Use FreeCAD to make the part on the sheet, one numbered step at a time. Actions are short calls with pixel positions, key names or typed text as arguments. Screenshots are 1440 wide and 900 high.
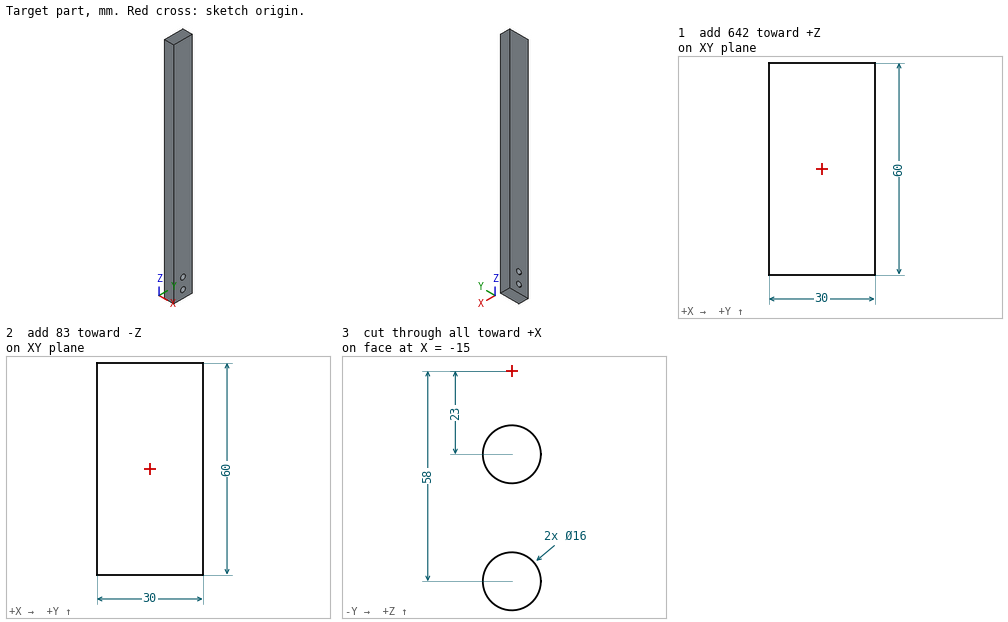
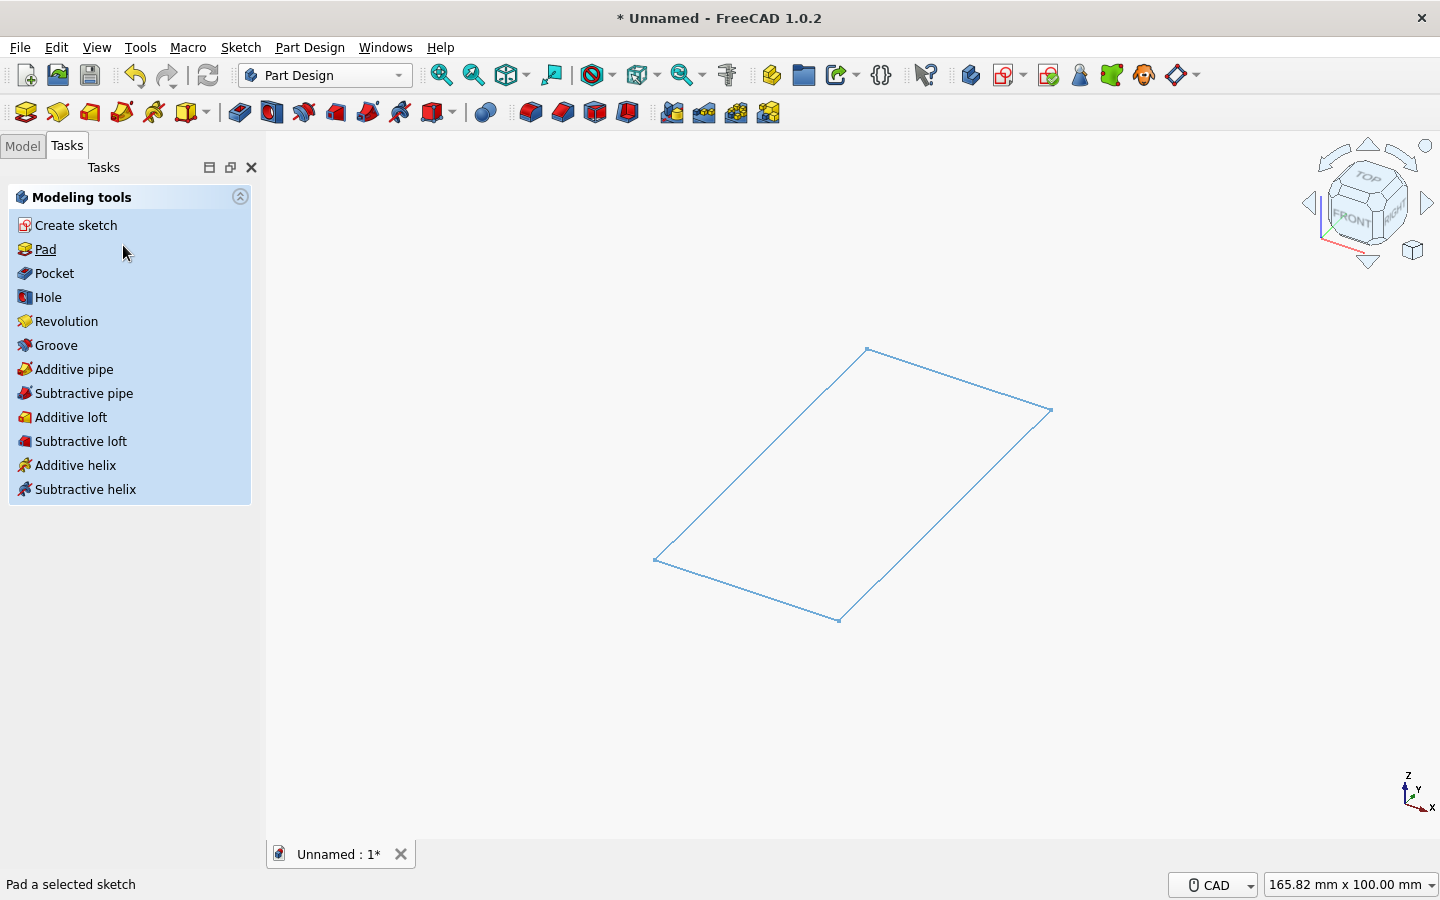
click(26, 112)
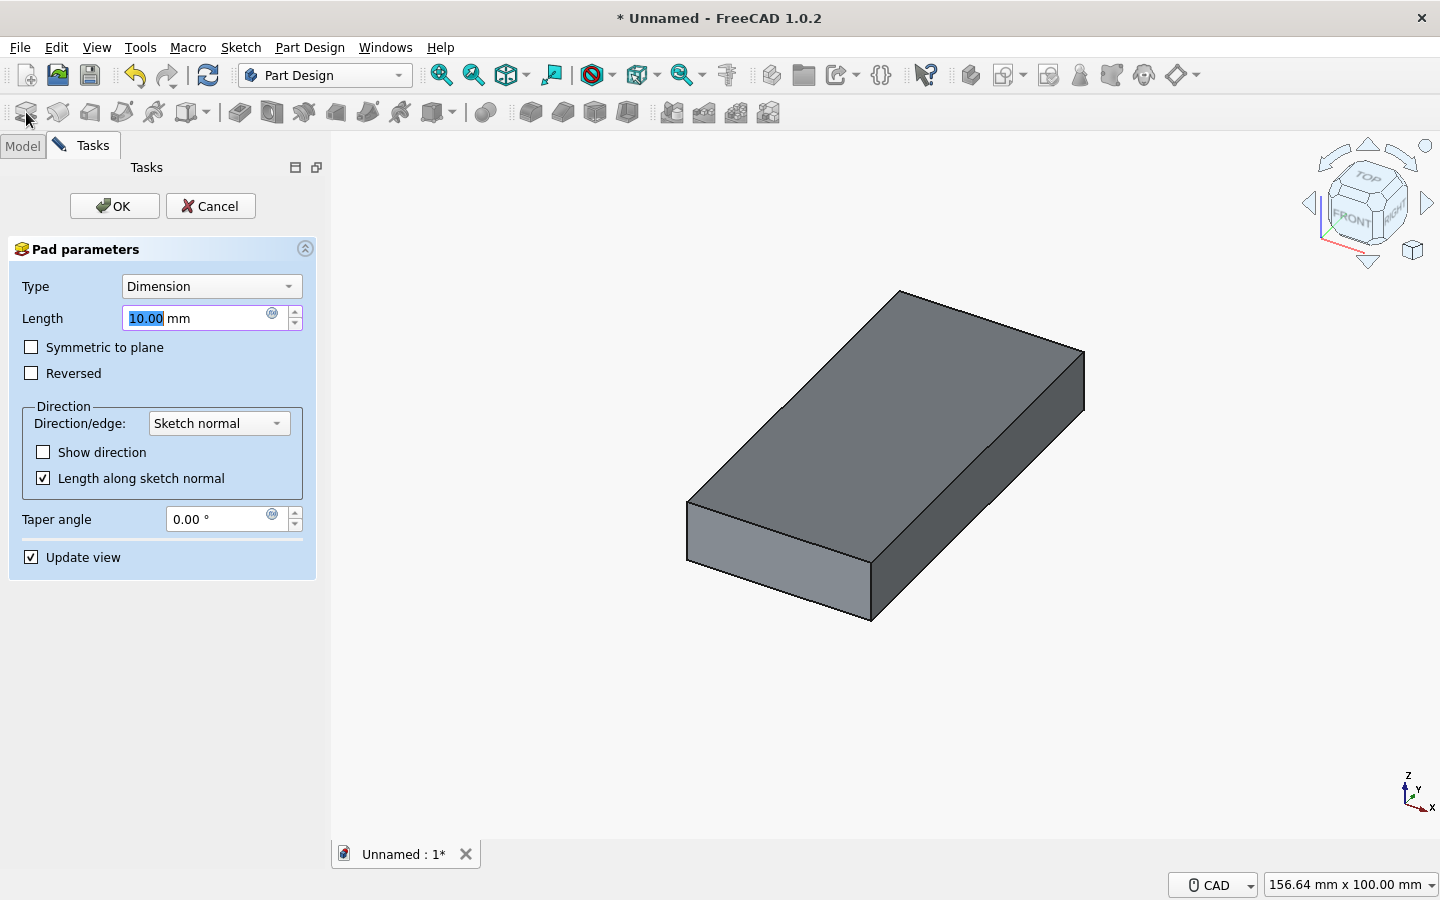
text(642)
key(Tab)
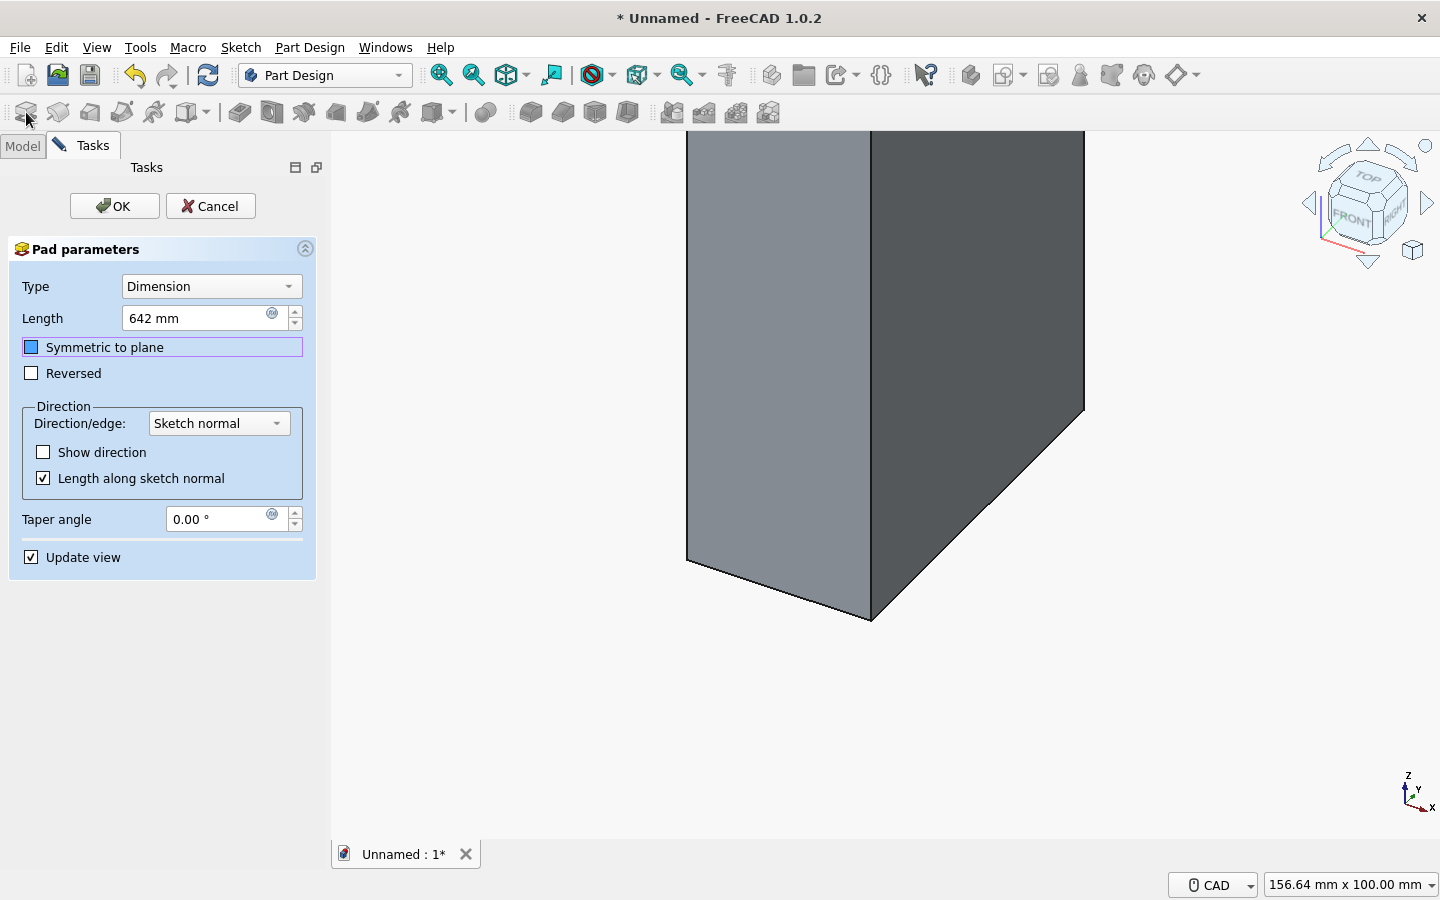
click(115, 206)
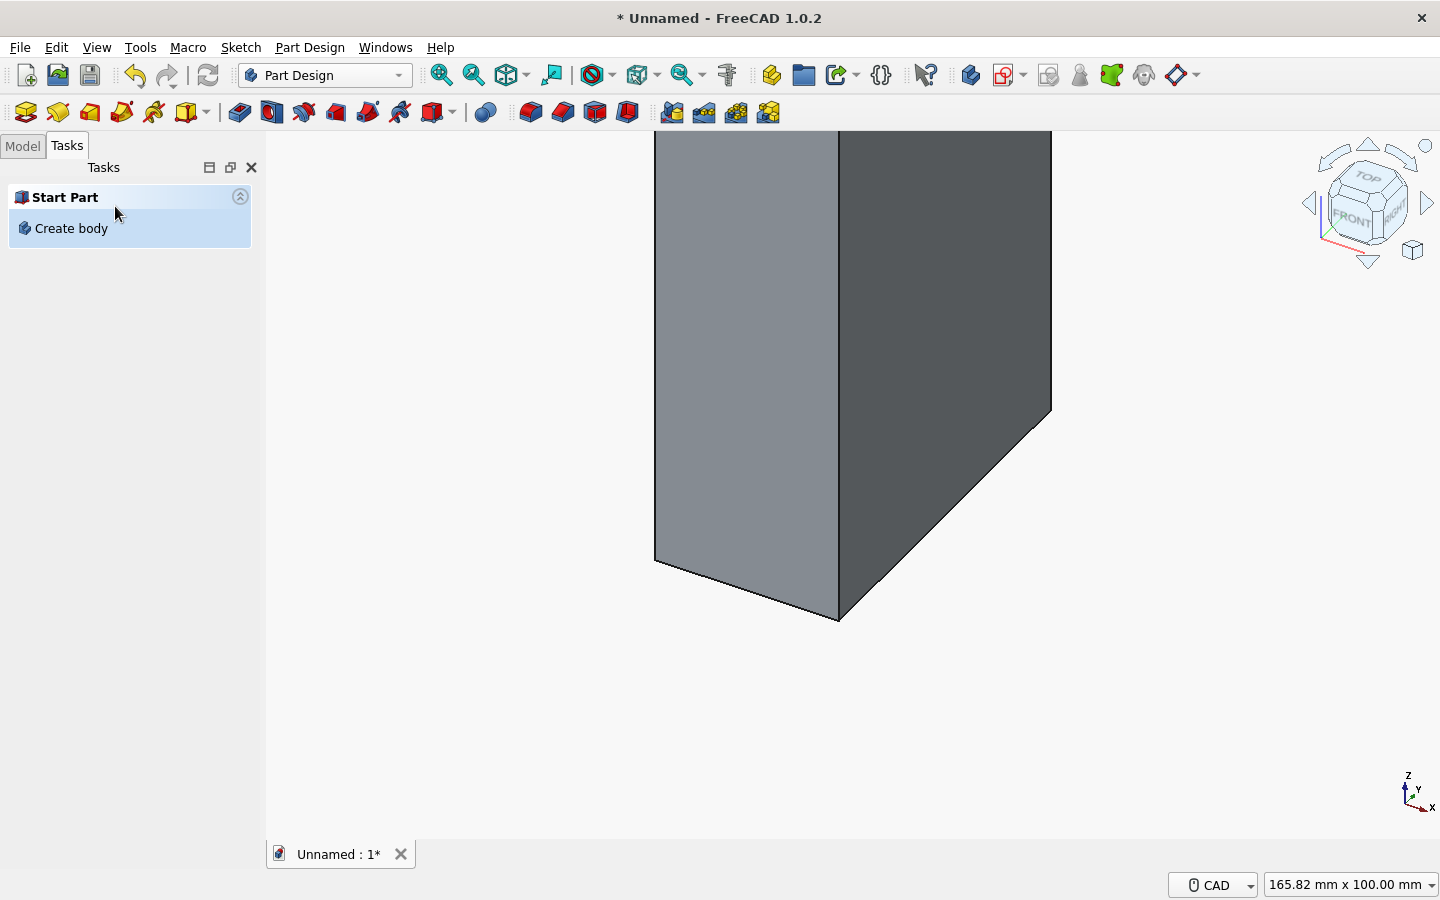
click(442, 76)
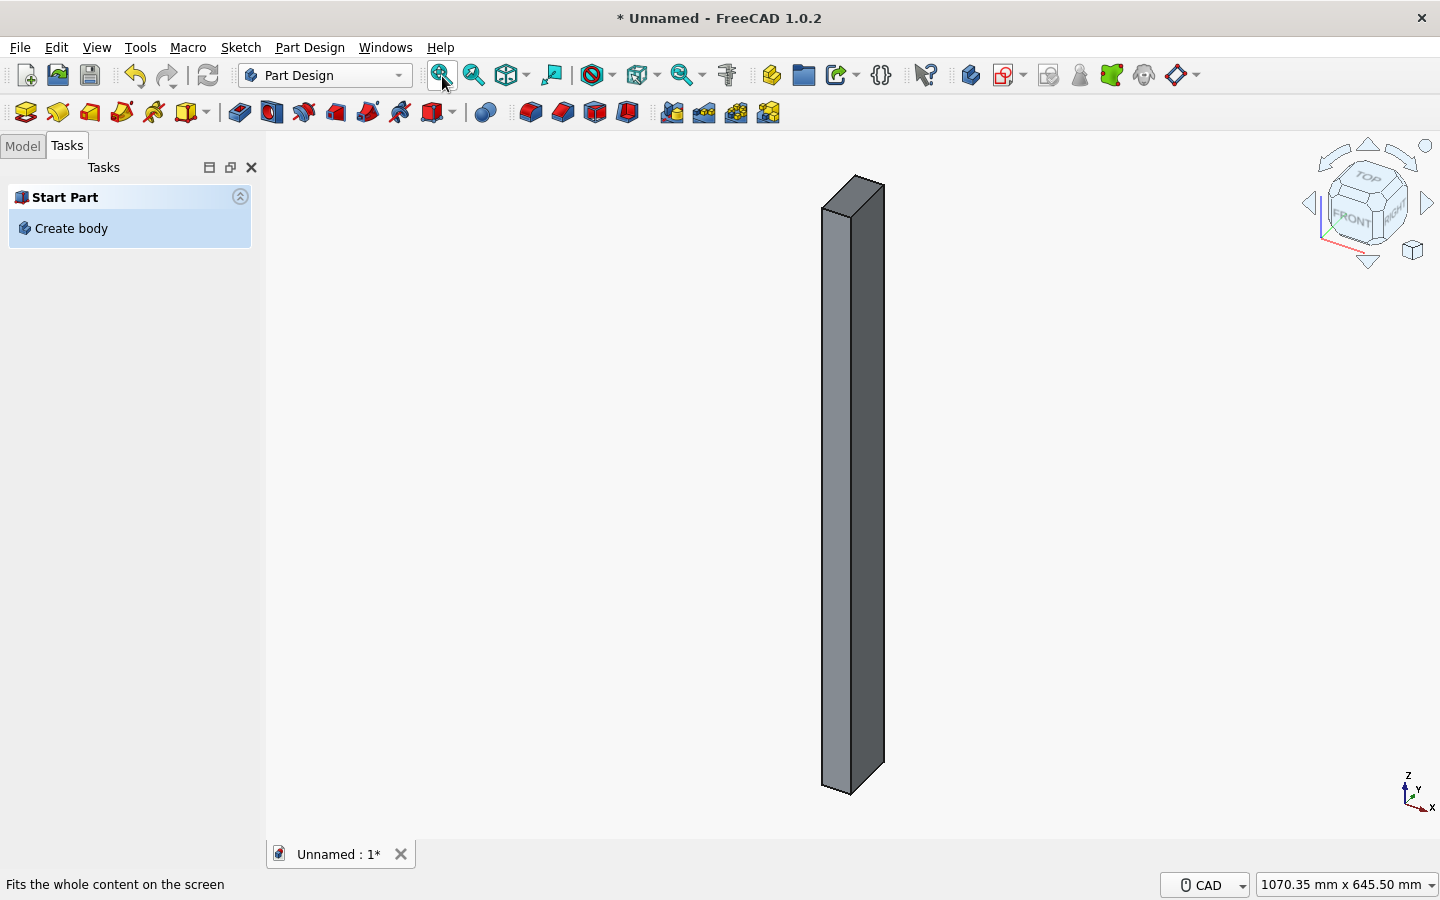
click(1004, 76)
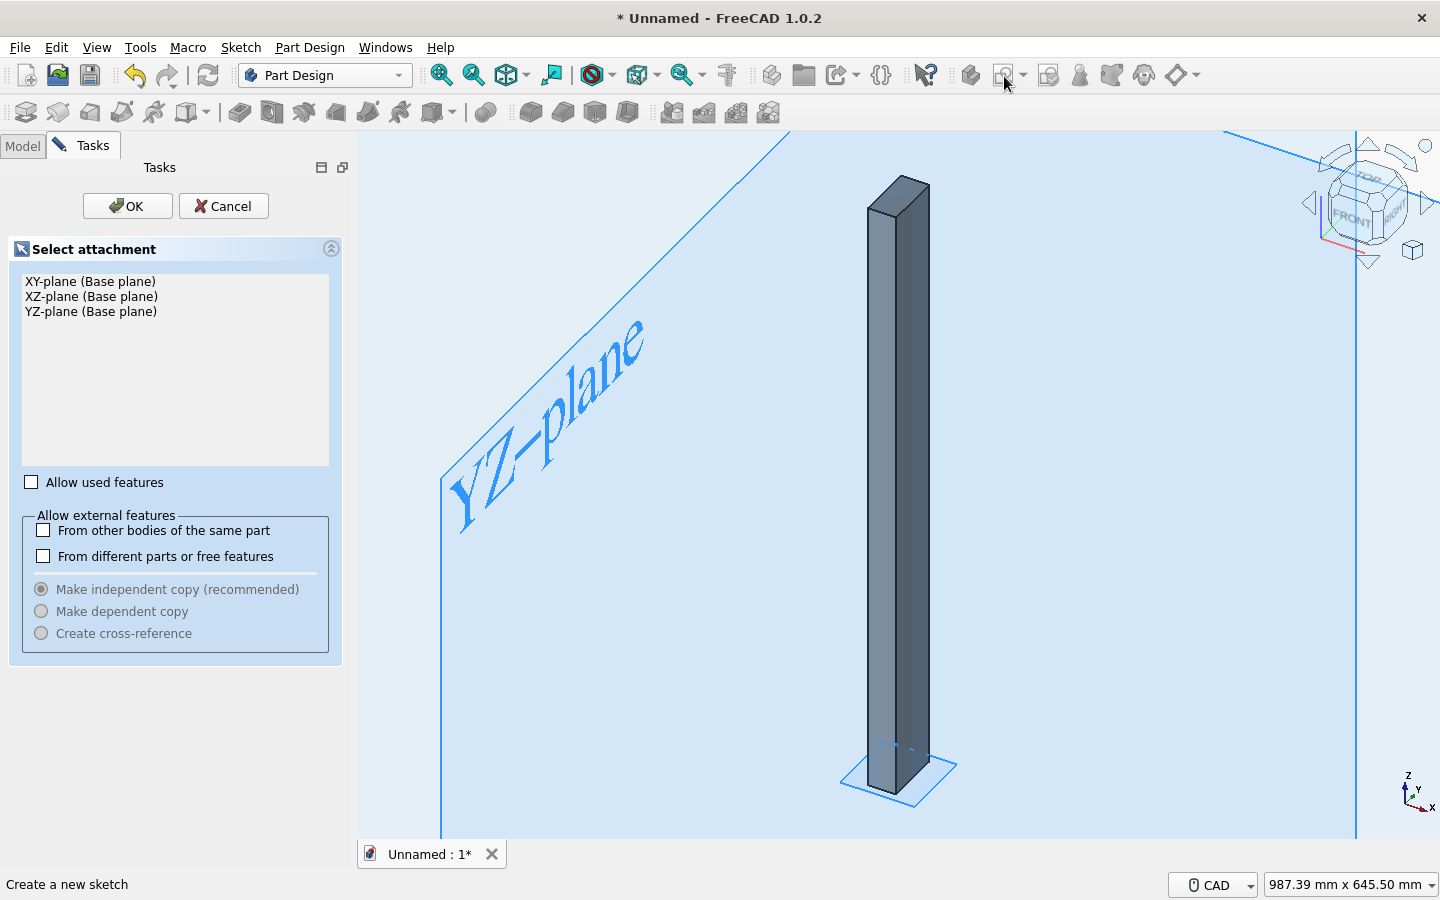
click(82, 282)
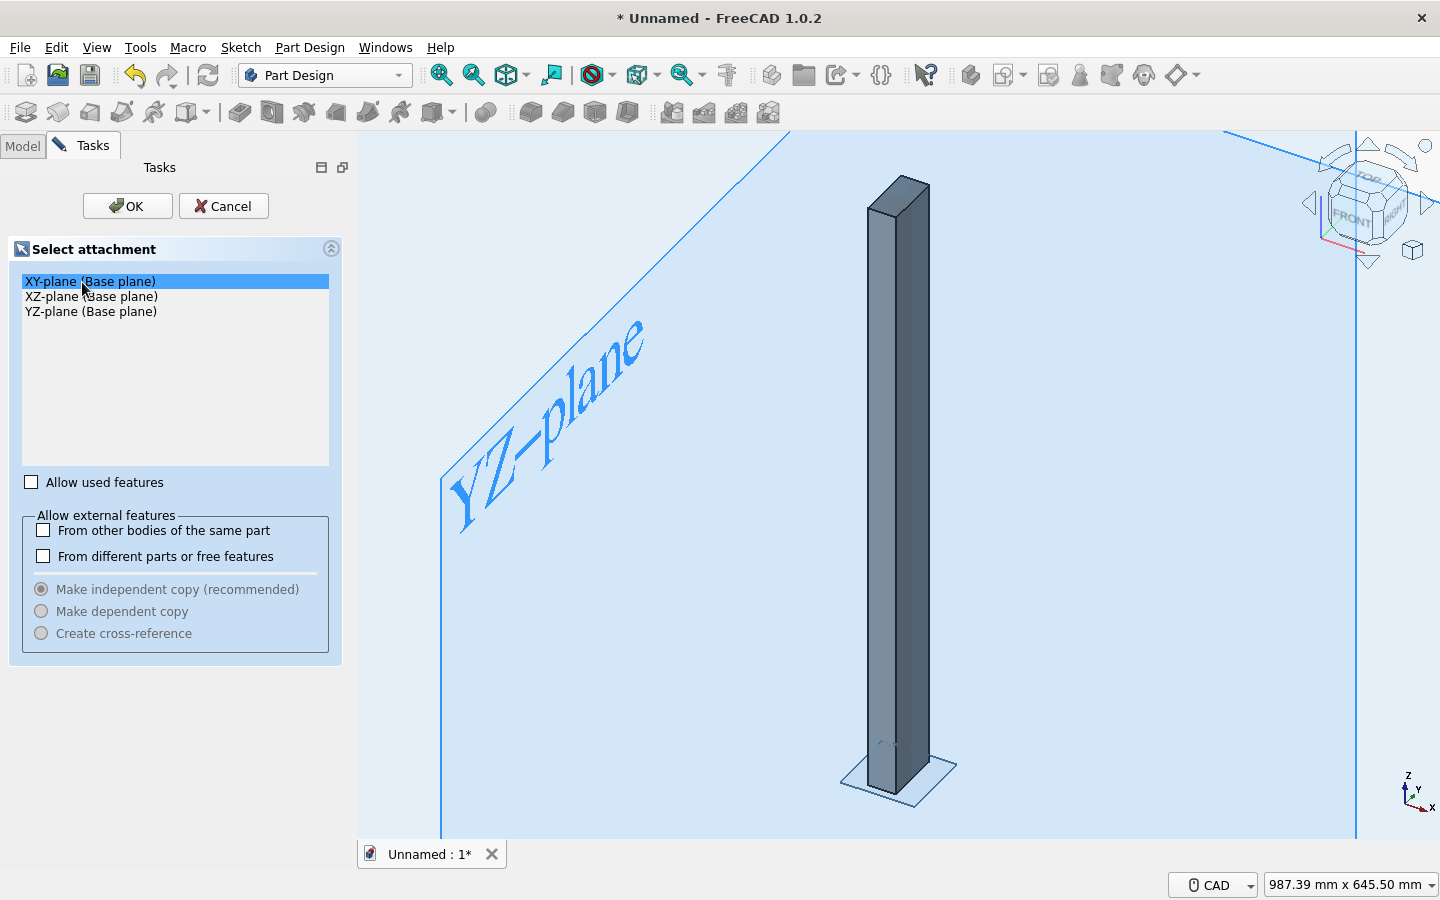
click(128, 206)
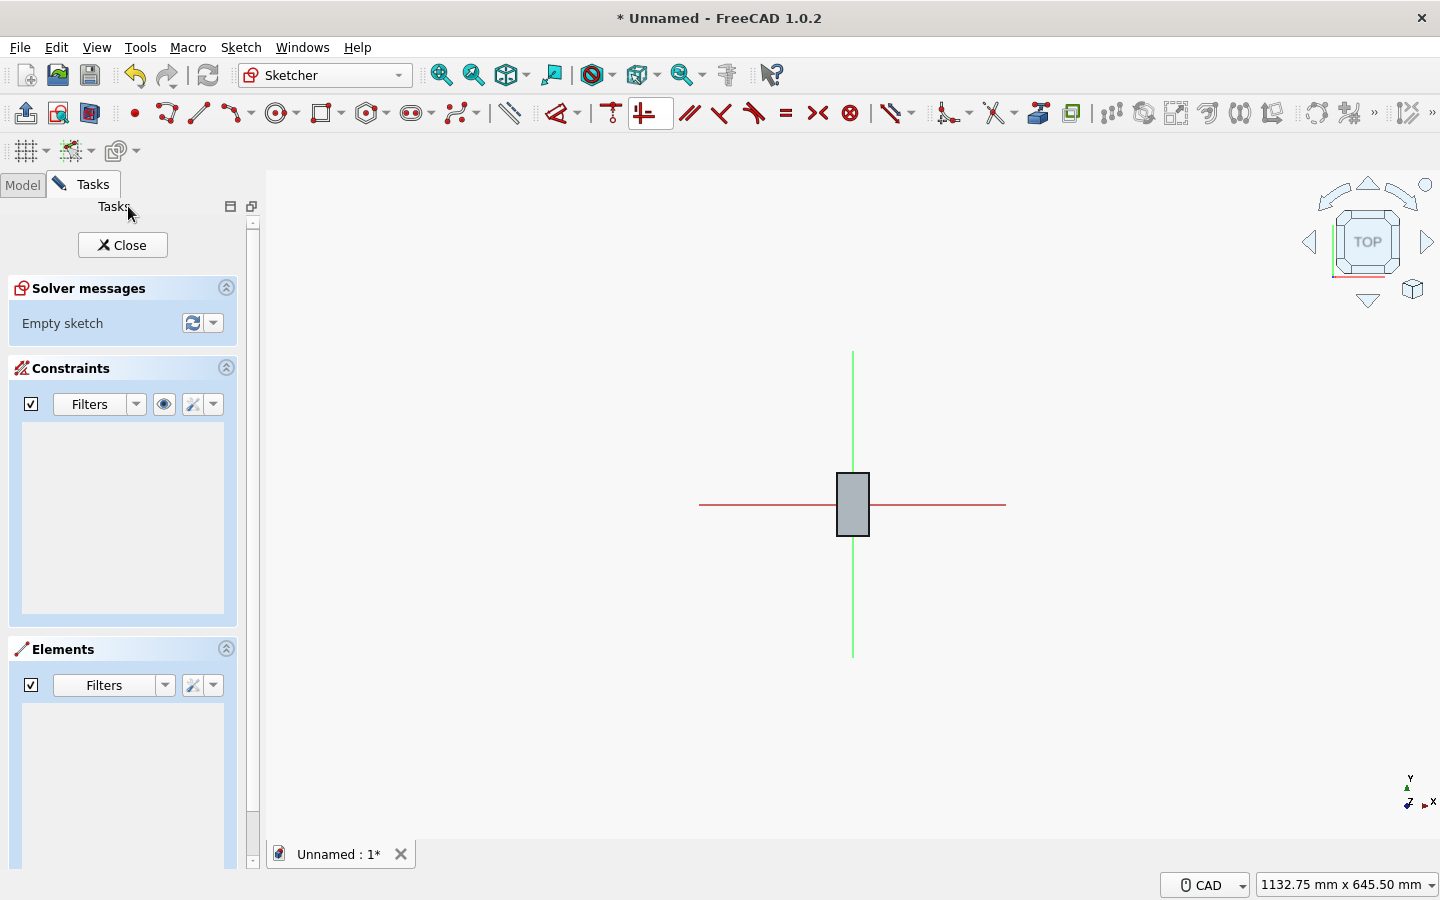
click(90, 114)